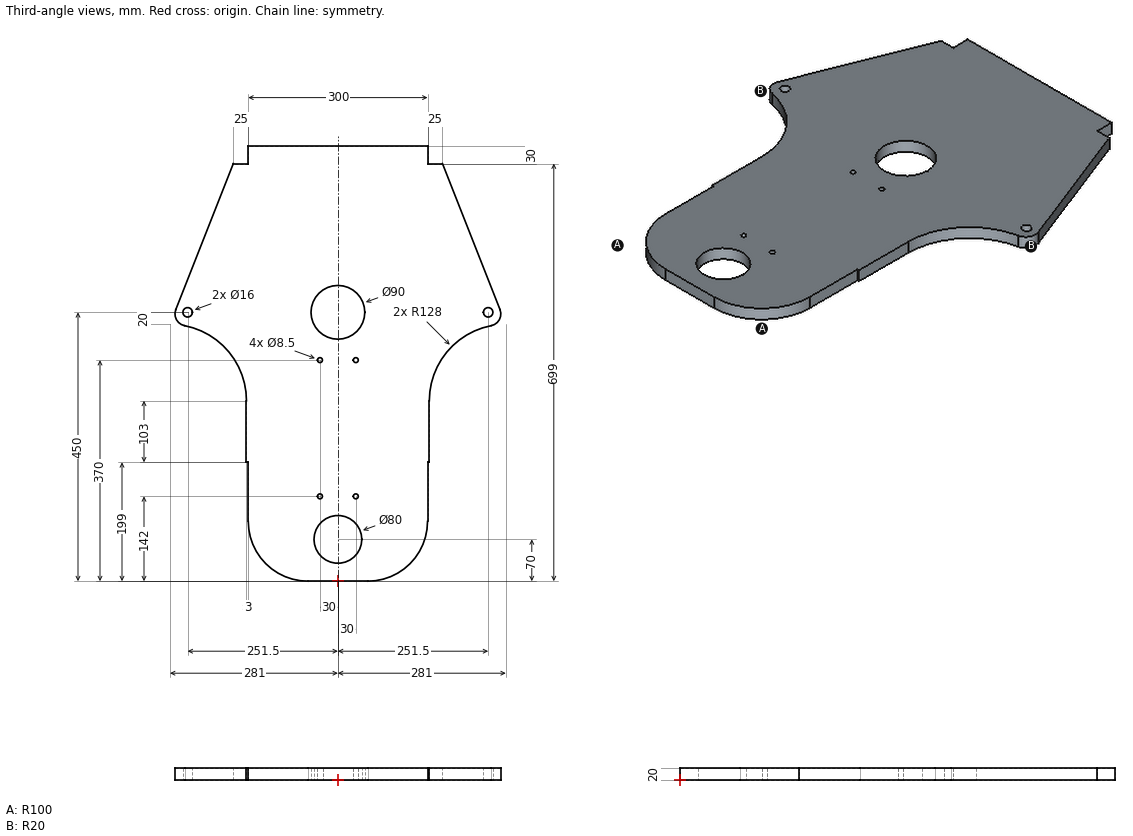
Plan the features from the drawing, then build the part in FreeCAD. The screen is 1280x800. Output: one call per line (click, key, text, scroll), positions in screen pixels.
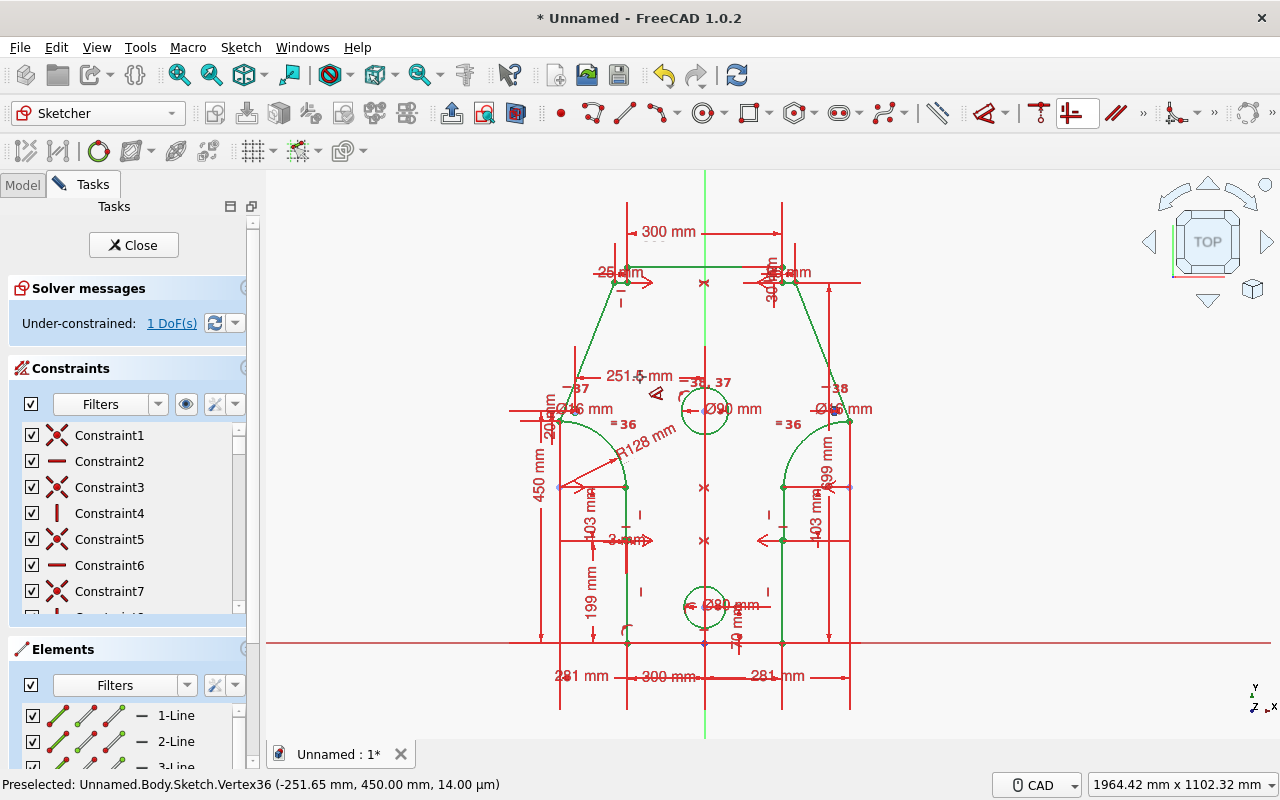
click(835, 411)
click(770, 377)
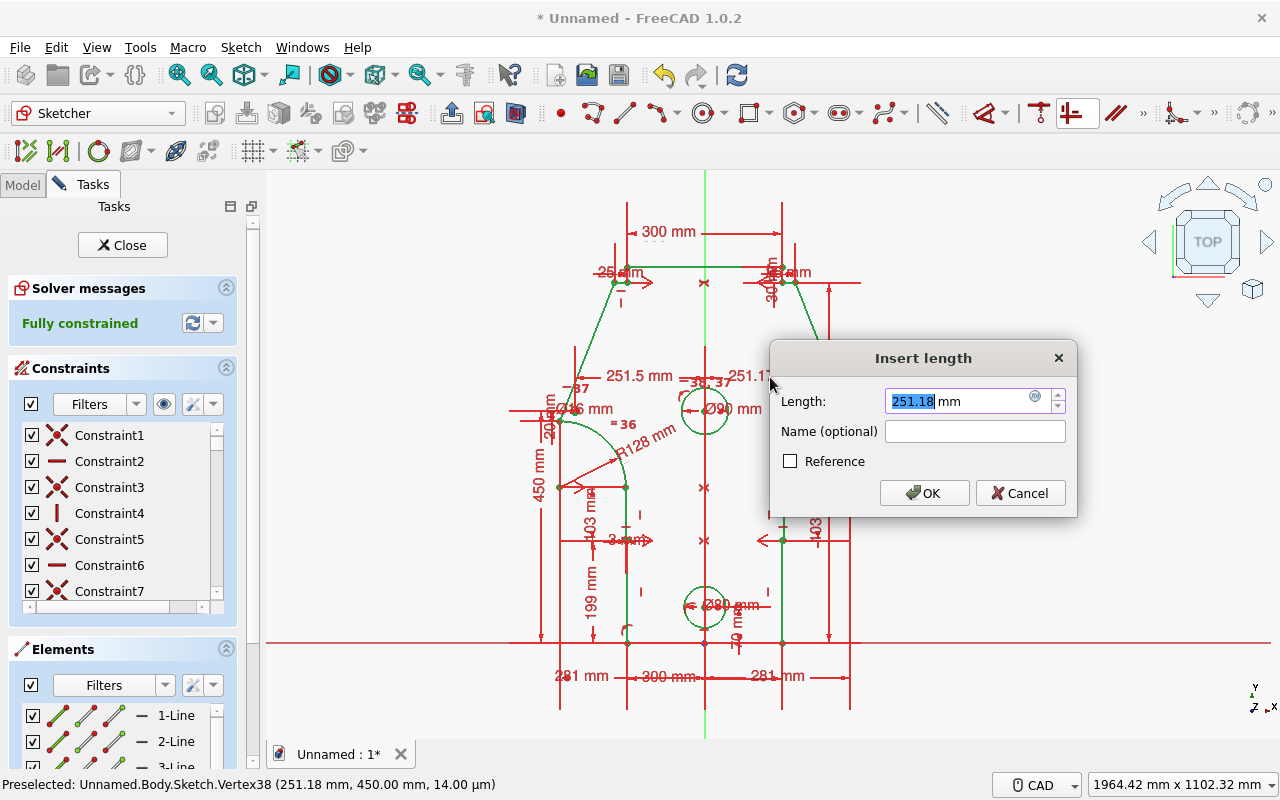
text(251.5)
key(Return)
key(Escape)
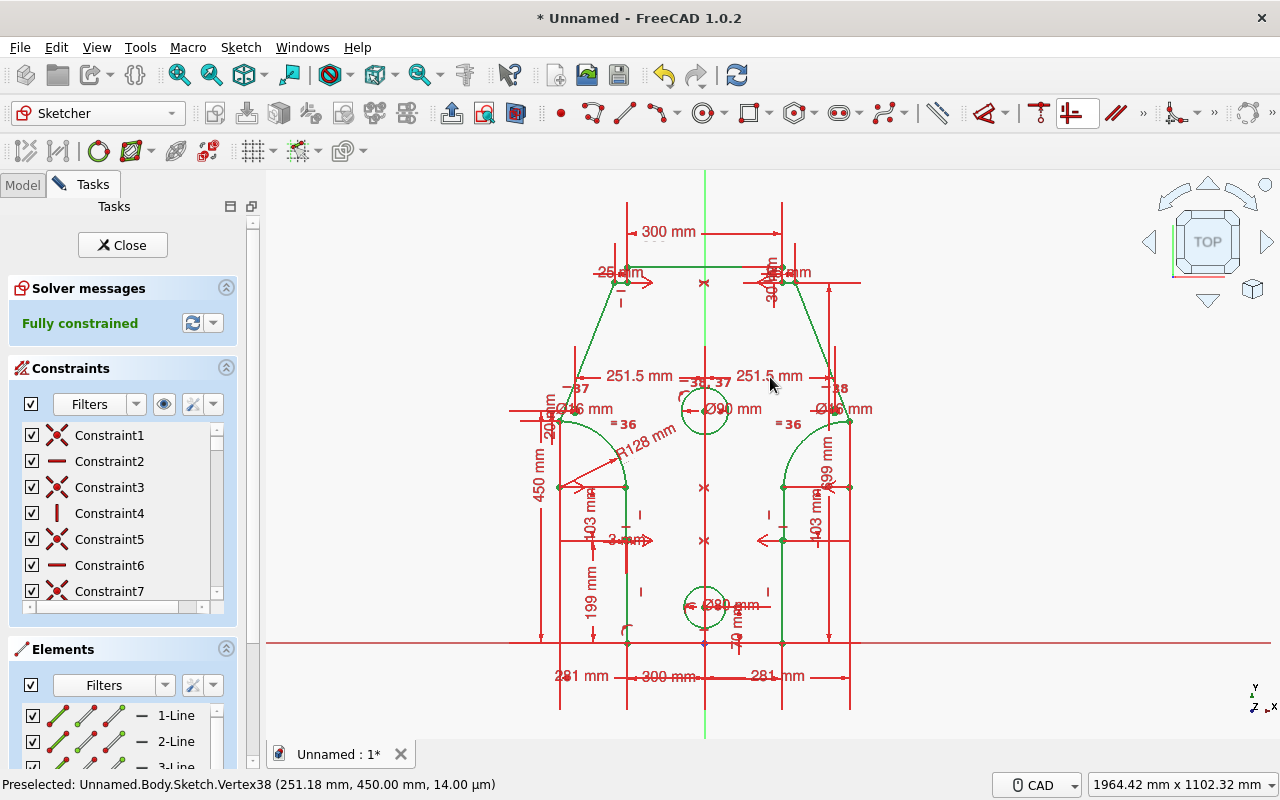
click(123, 245)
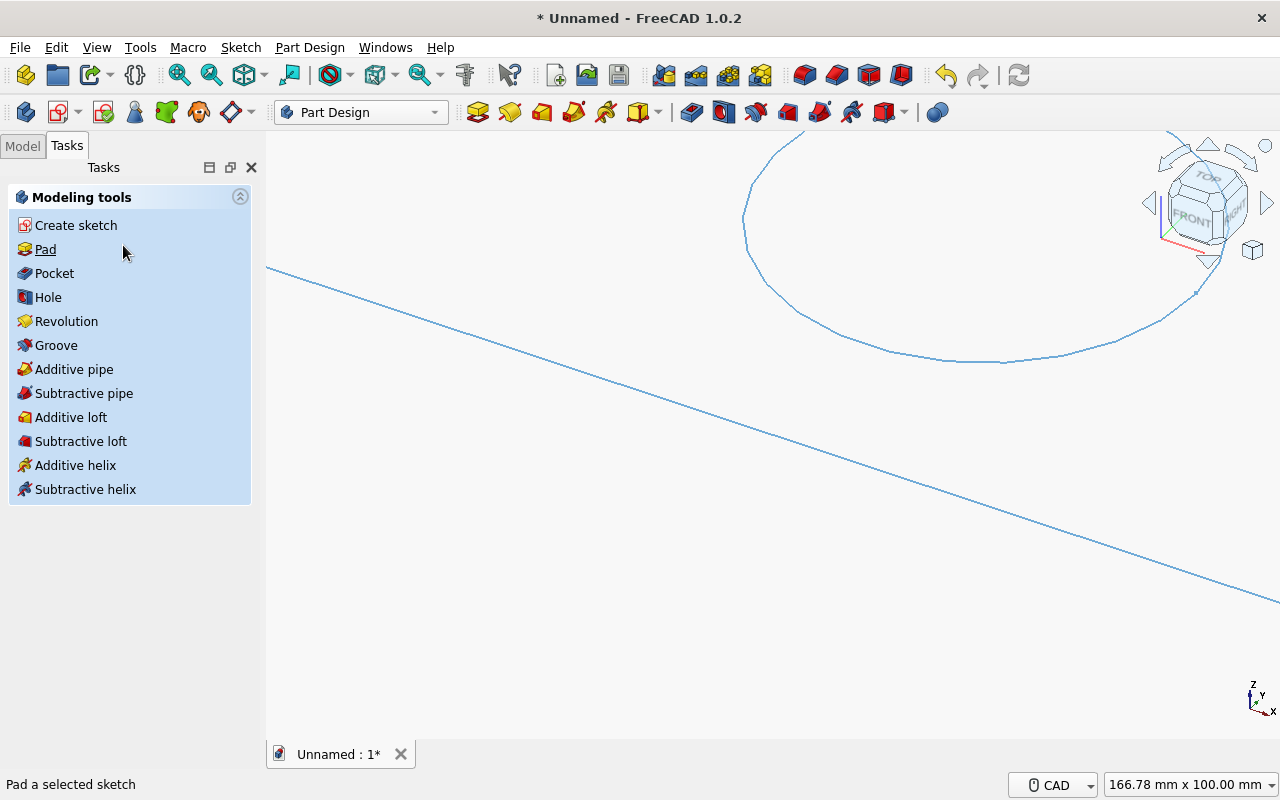
click(478, 112)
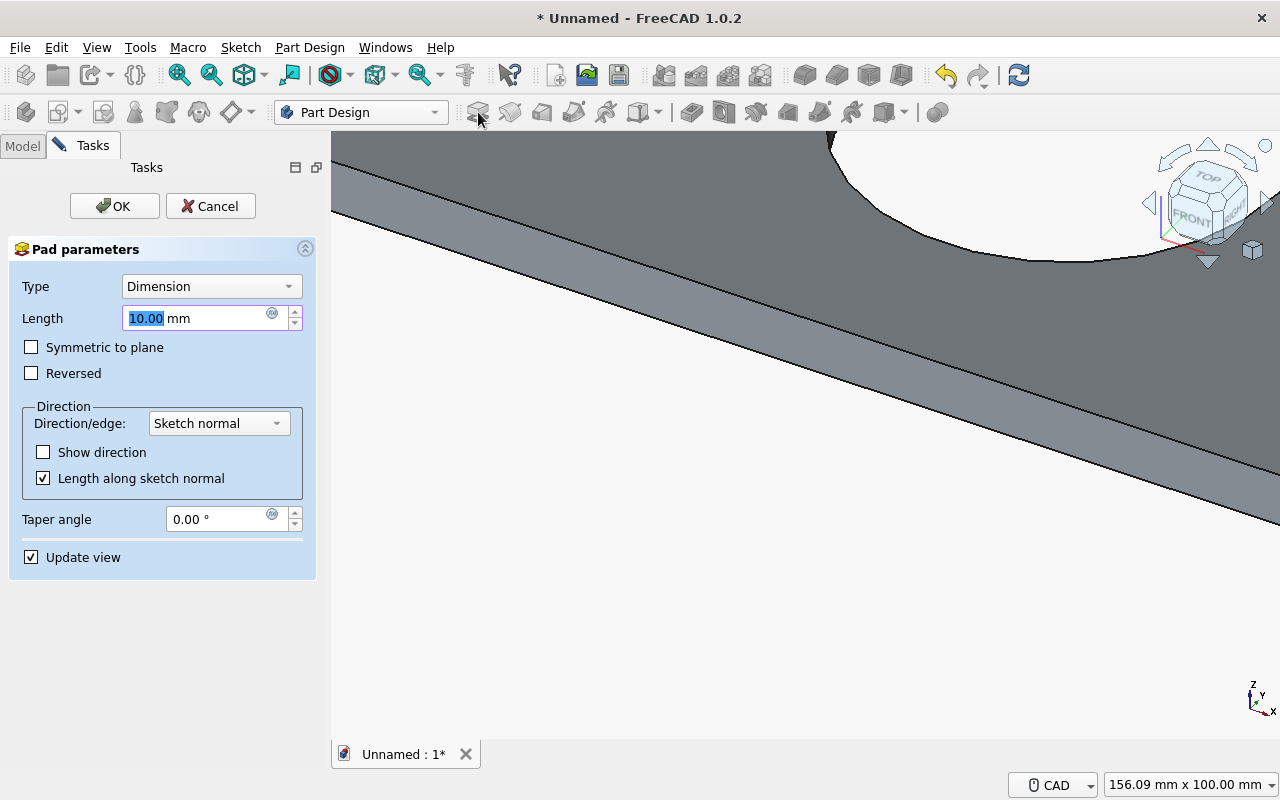
text(20)
key(Tab)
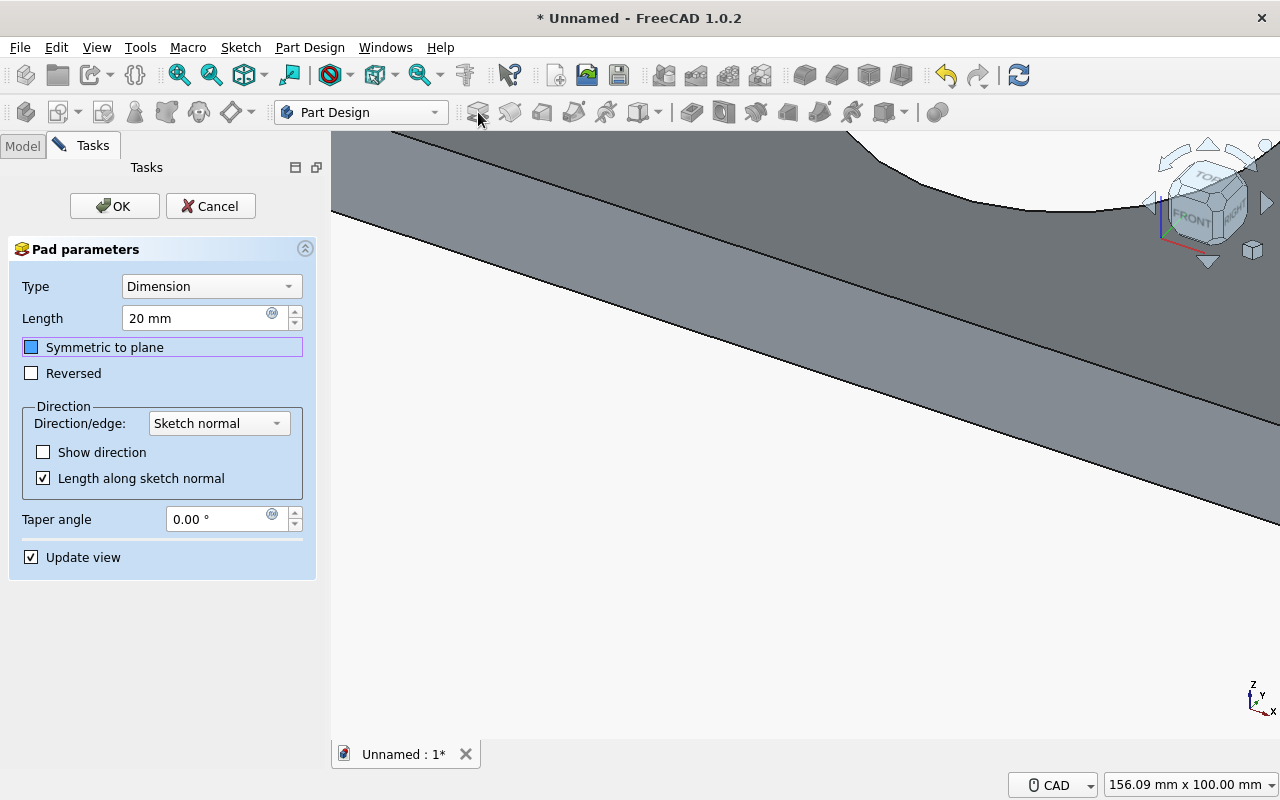
click(115, 206)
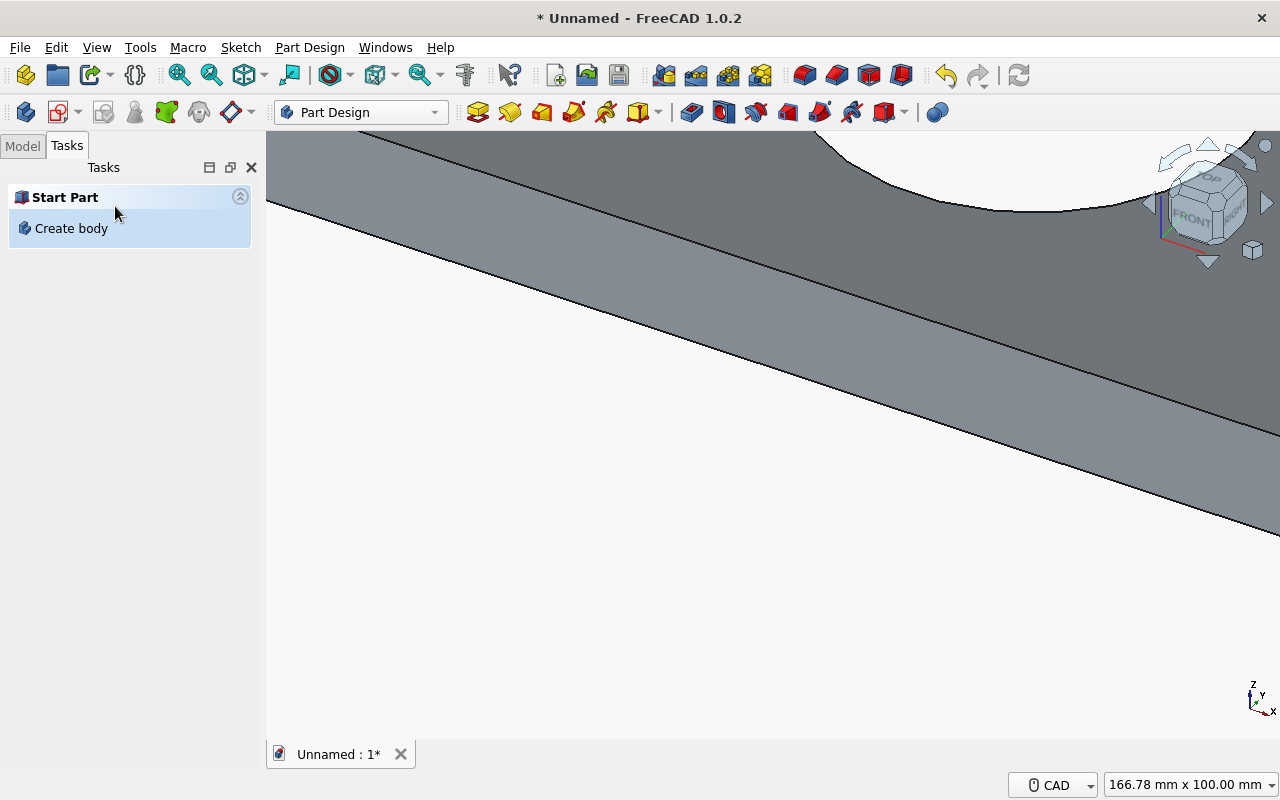
click(180, 76)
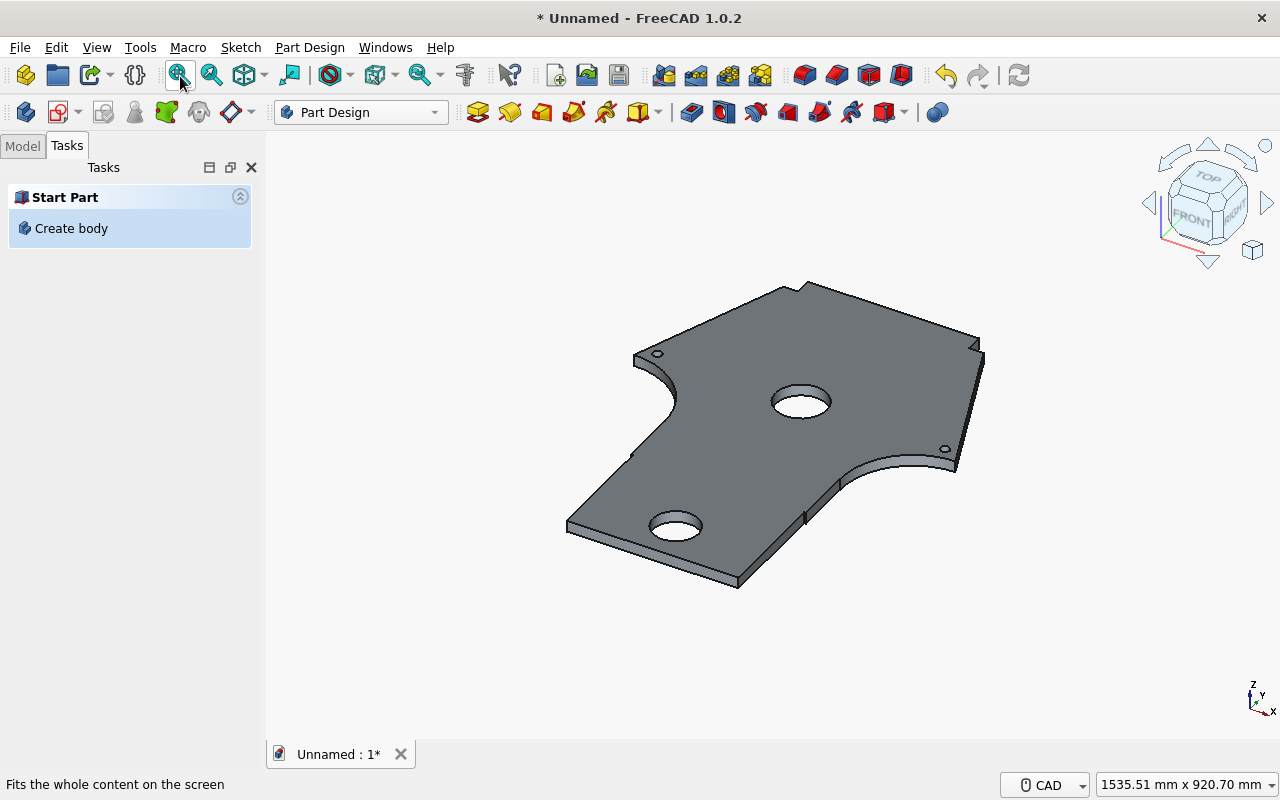
click(738, 583)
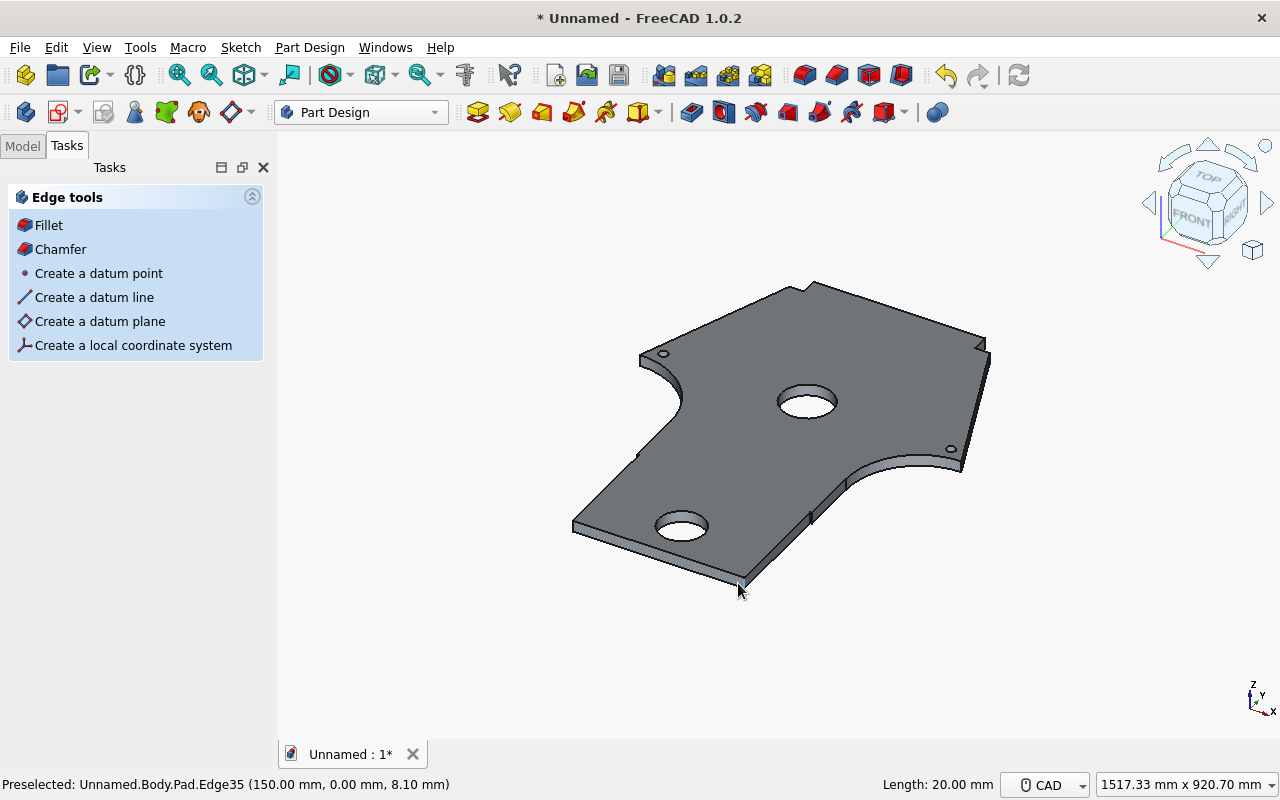
scroll(573, 525, up, 6)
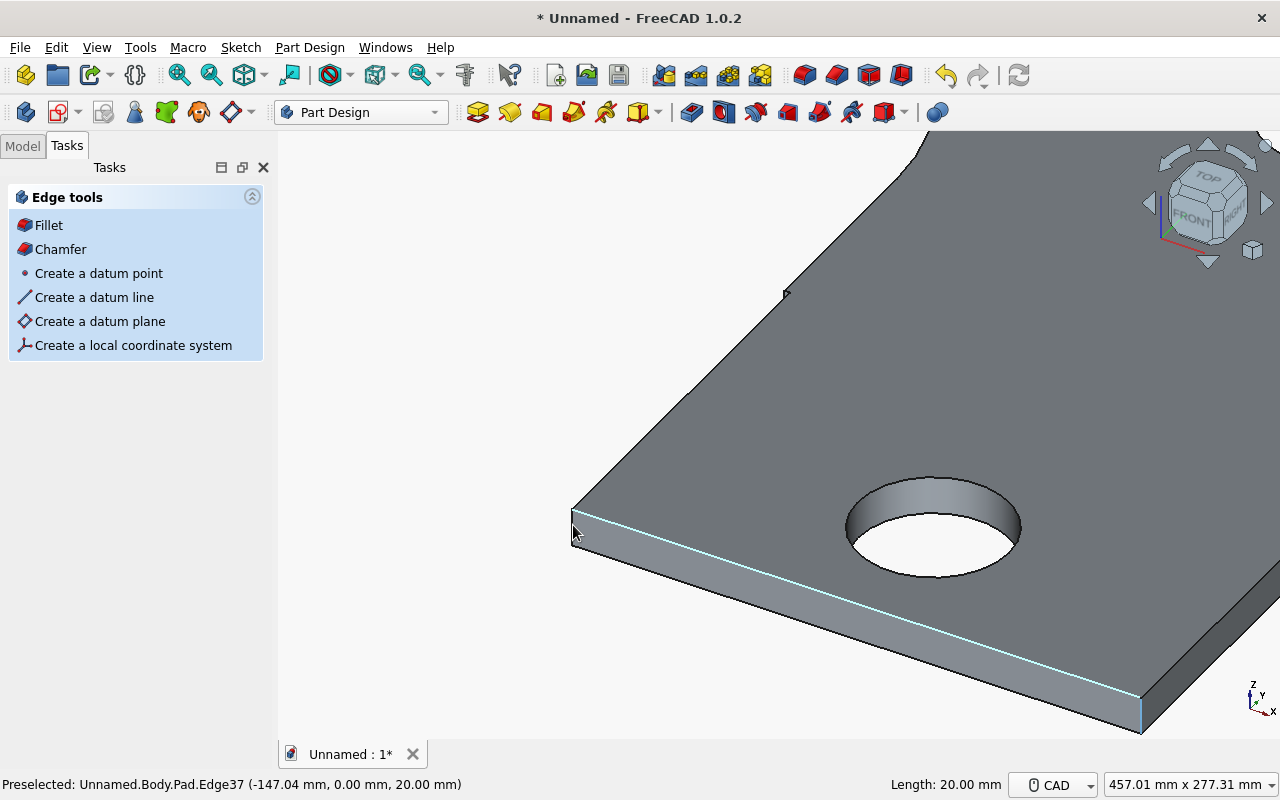
click(180, 76)